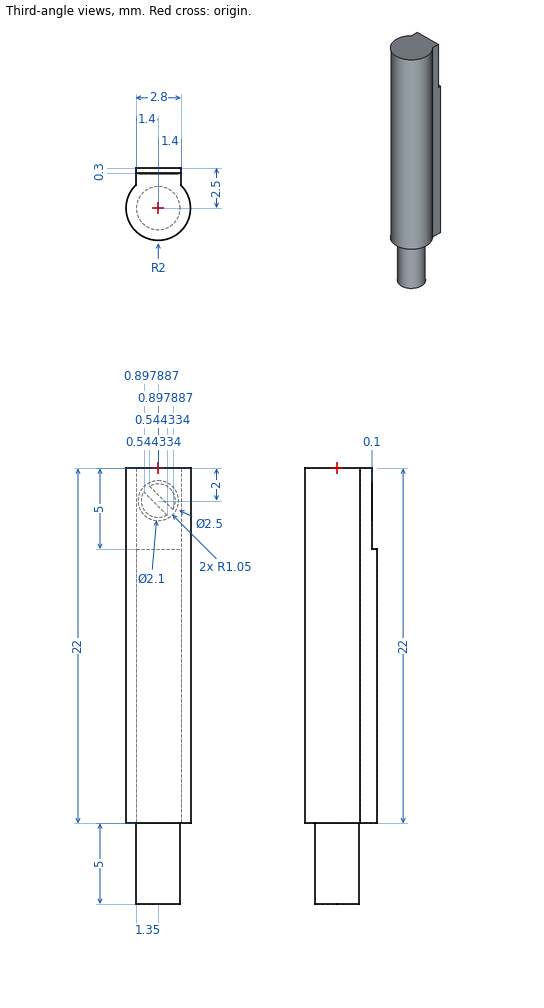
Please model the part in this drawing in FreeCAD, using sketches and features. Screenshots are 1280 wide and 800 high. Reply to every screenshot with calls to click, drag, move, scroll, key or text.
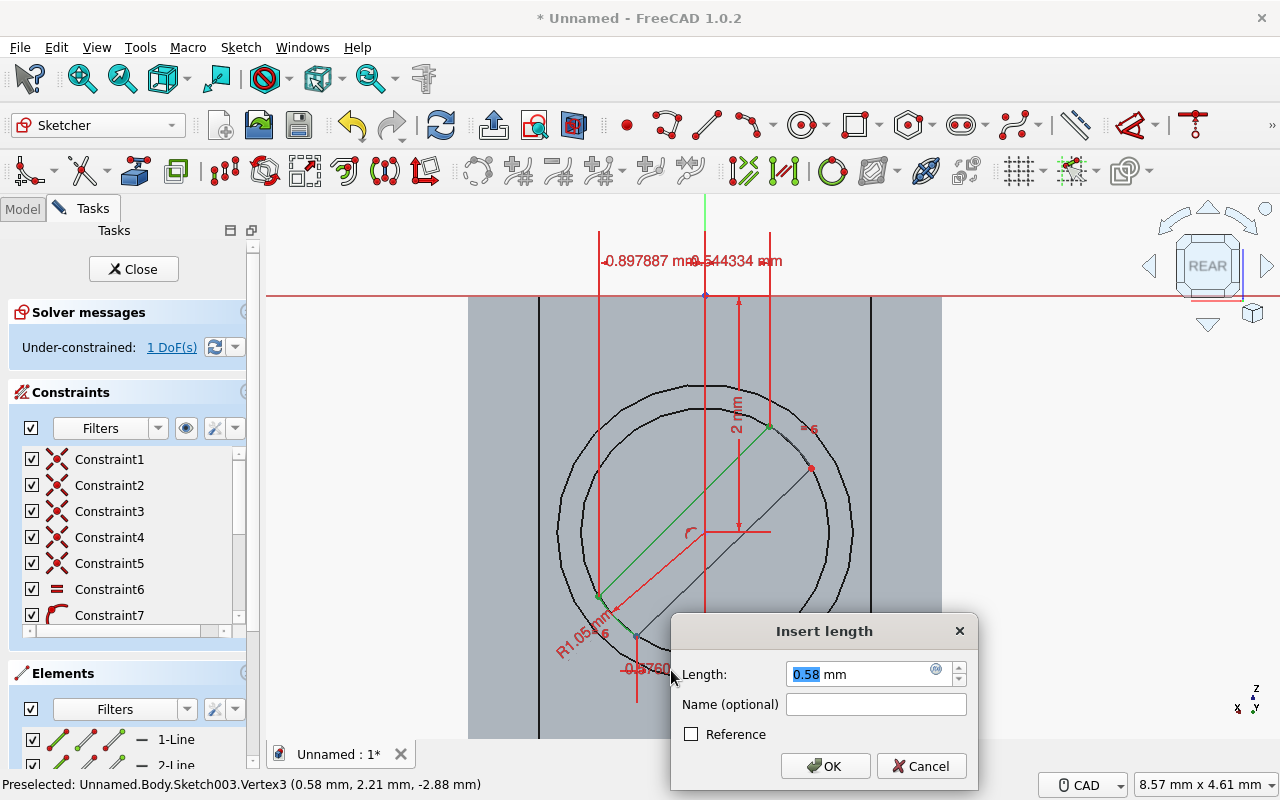
text(0.544334)
key(Return)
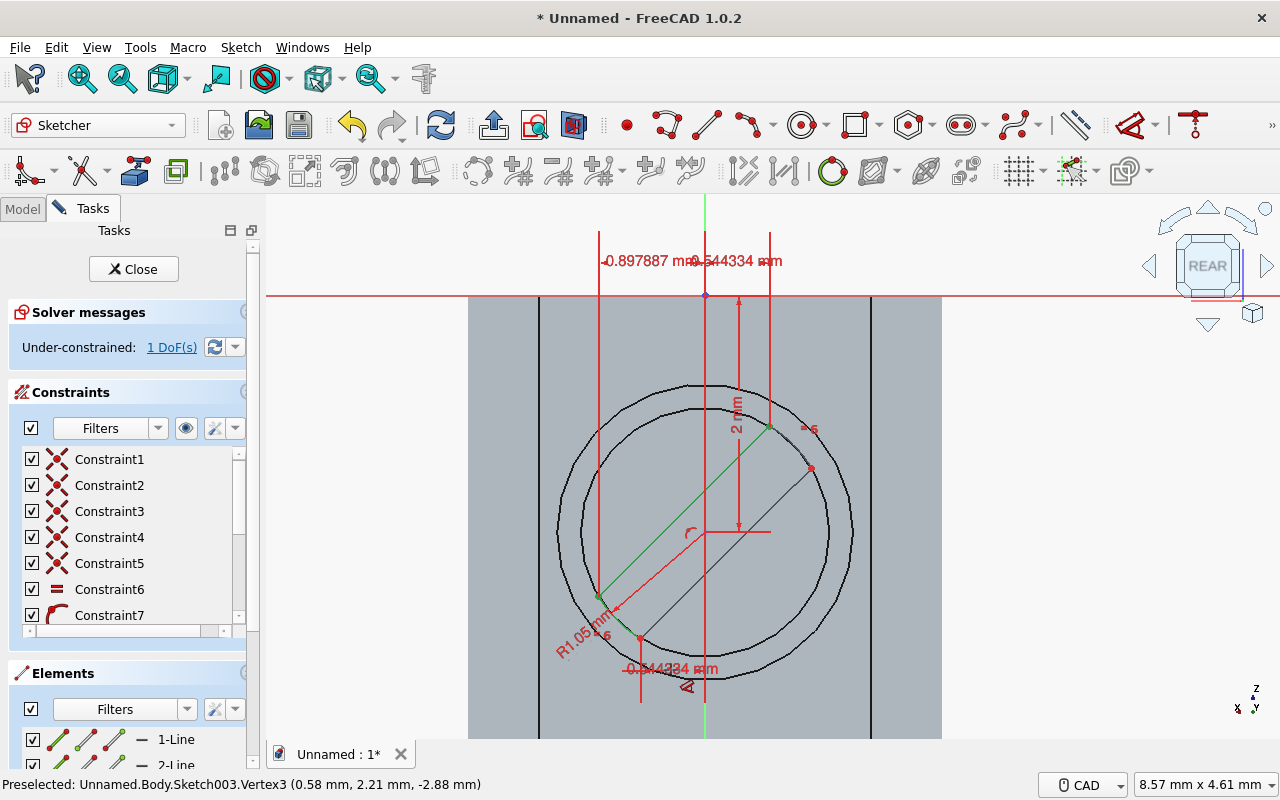
click(812, 468)
click(758, 502)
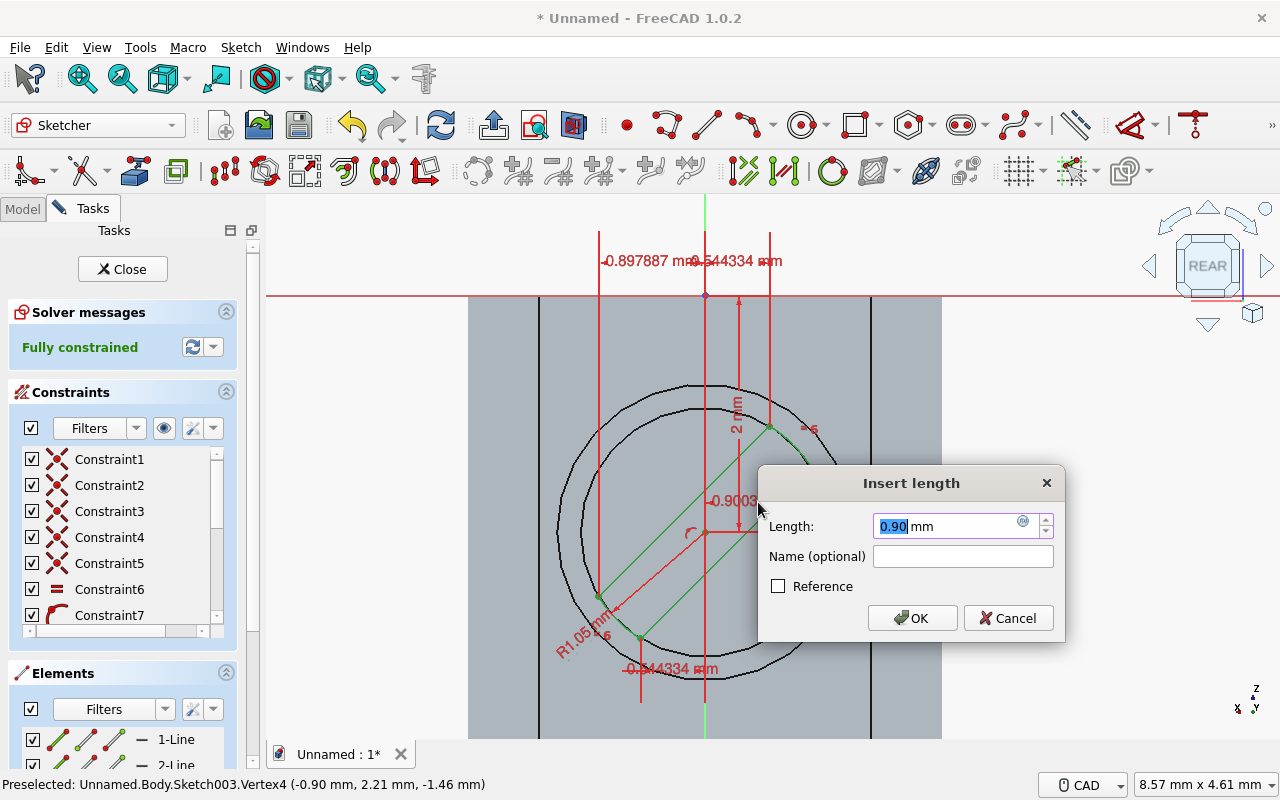
text(0.897887)
key(Return)
key(Escape)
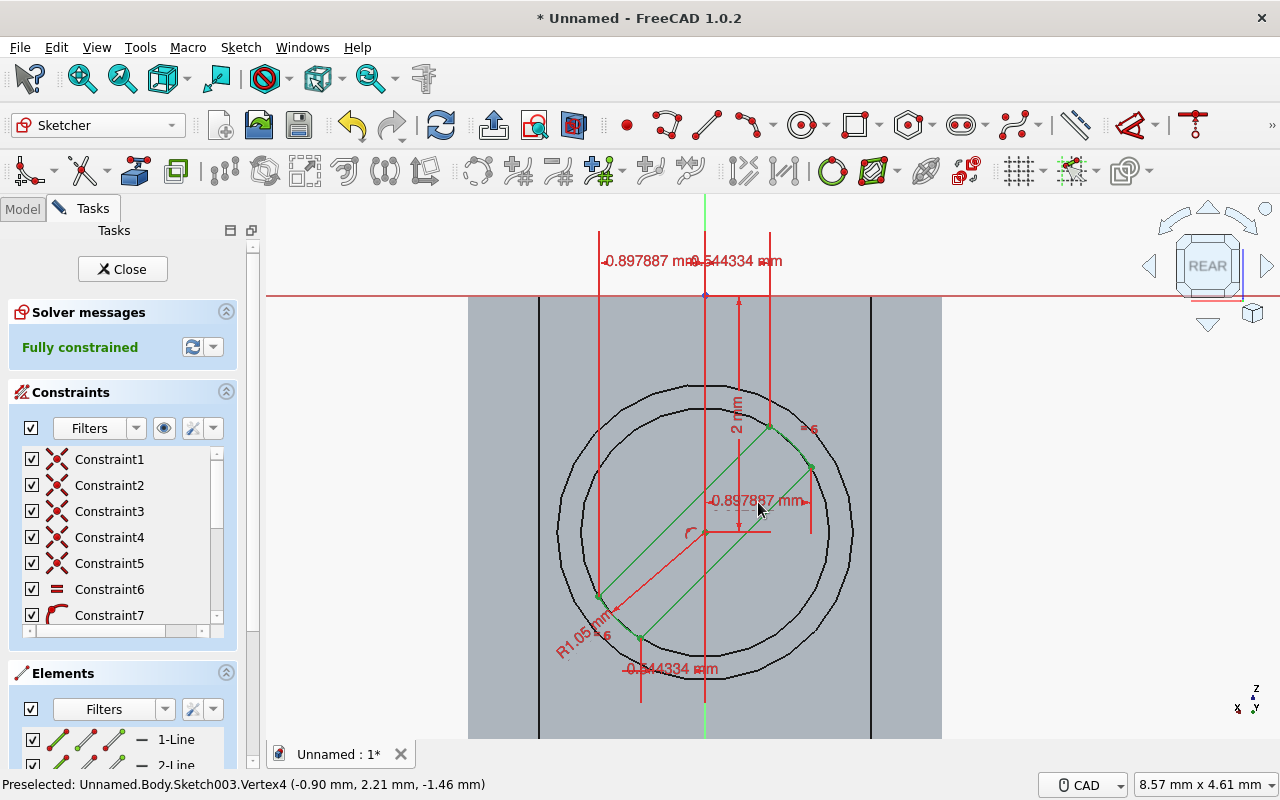
click(123, 269)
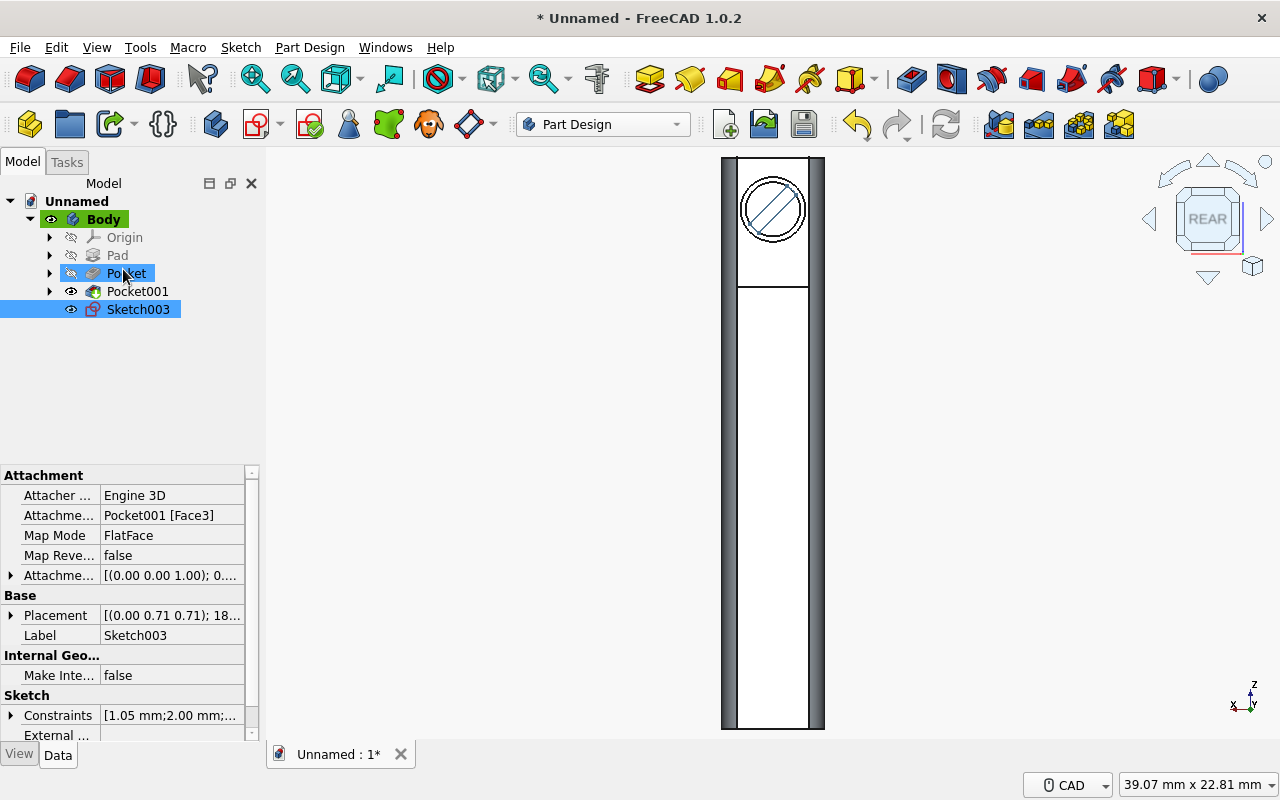
click(912, 80)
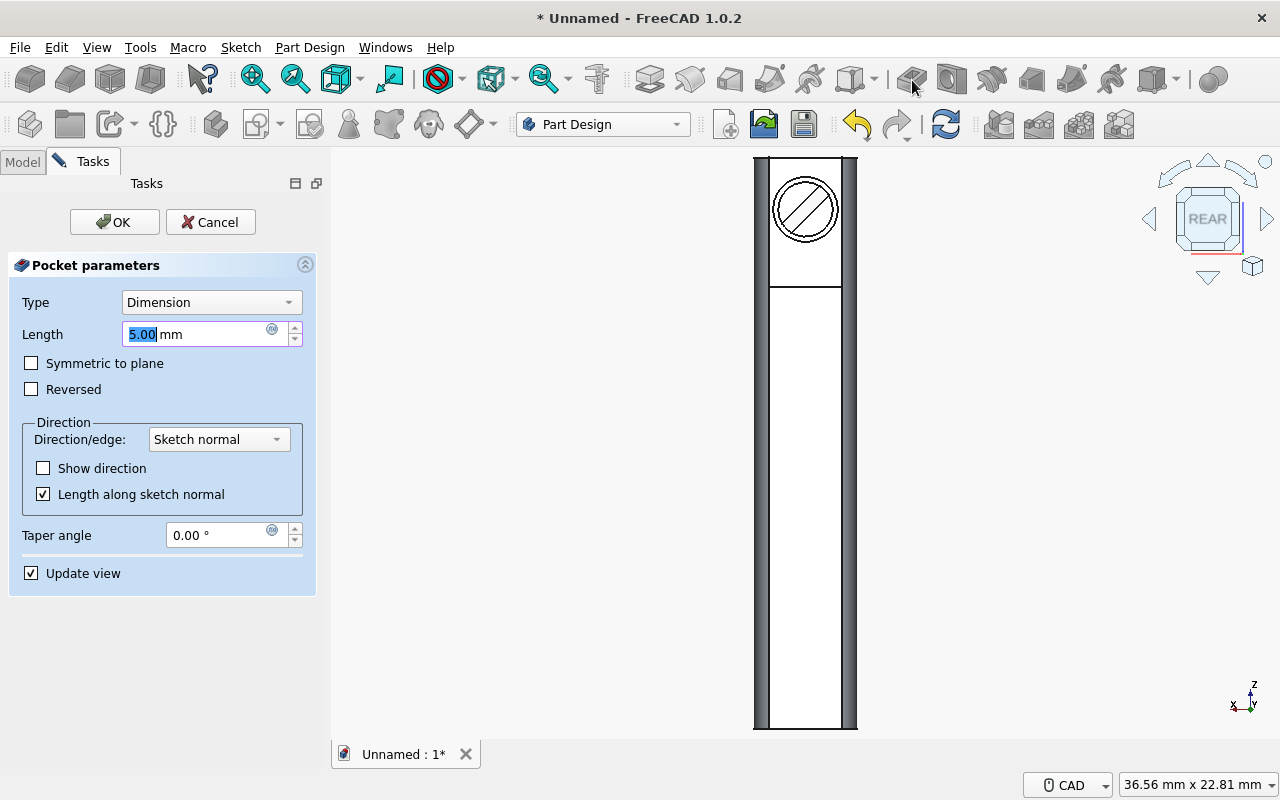
text(0.1)
key(Tab)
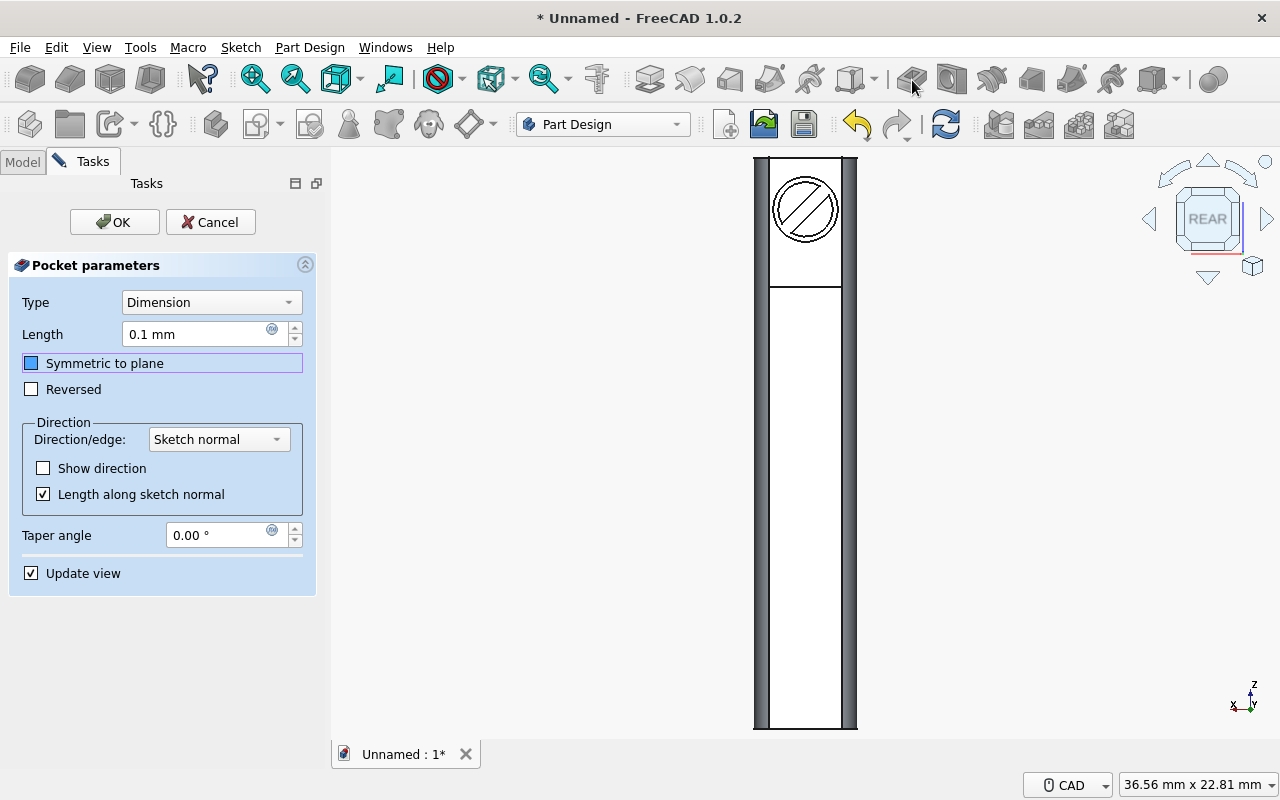
click(115, 222)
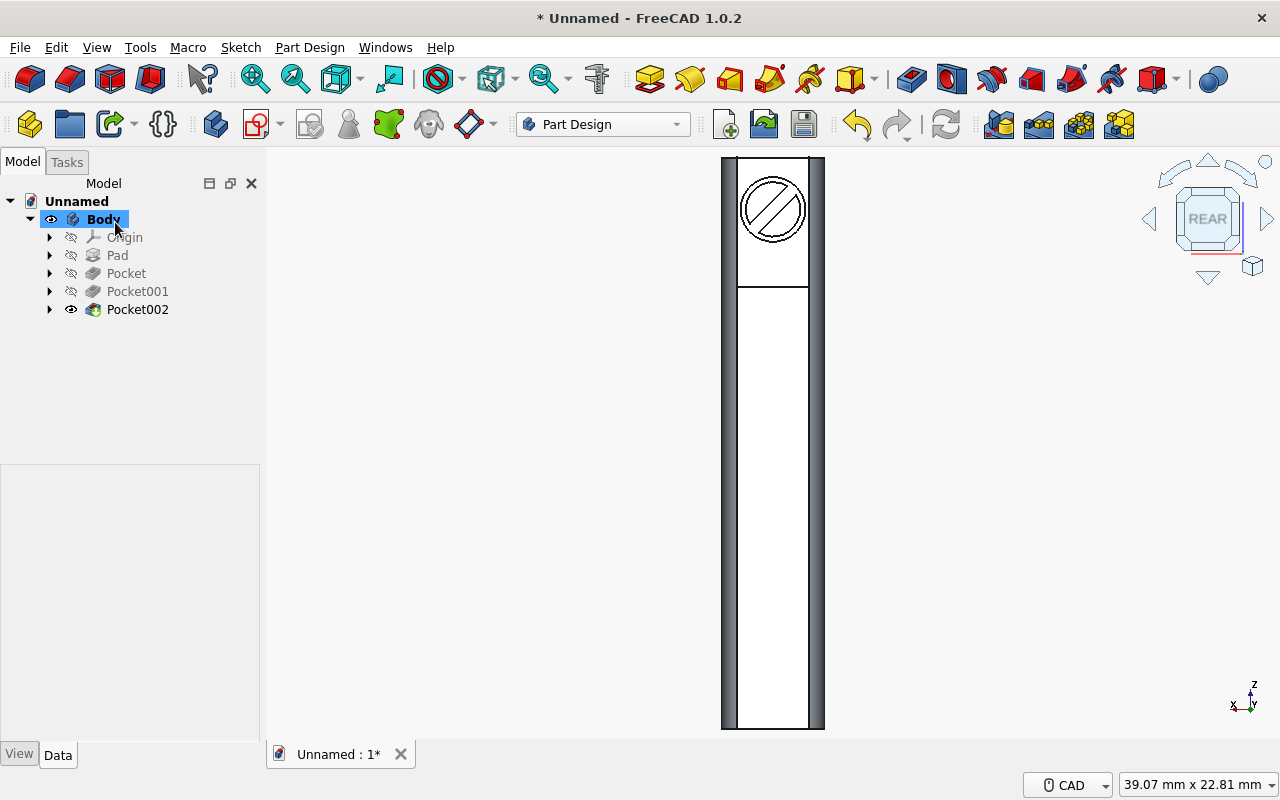
click(256, 124)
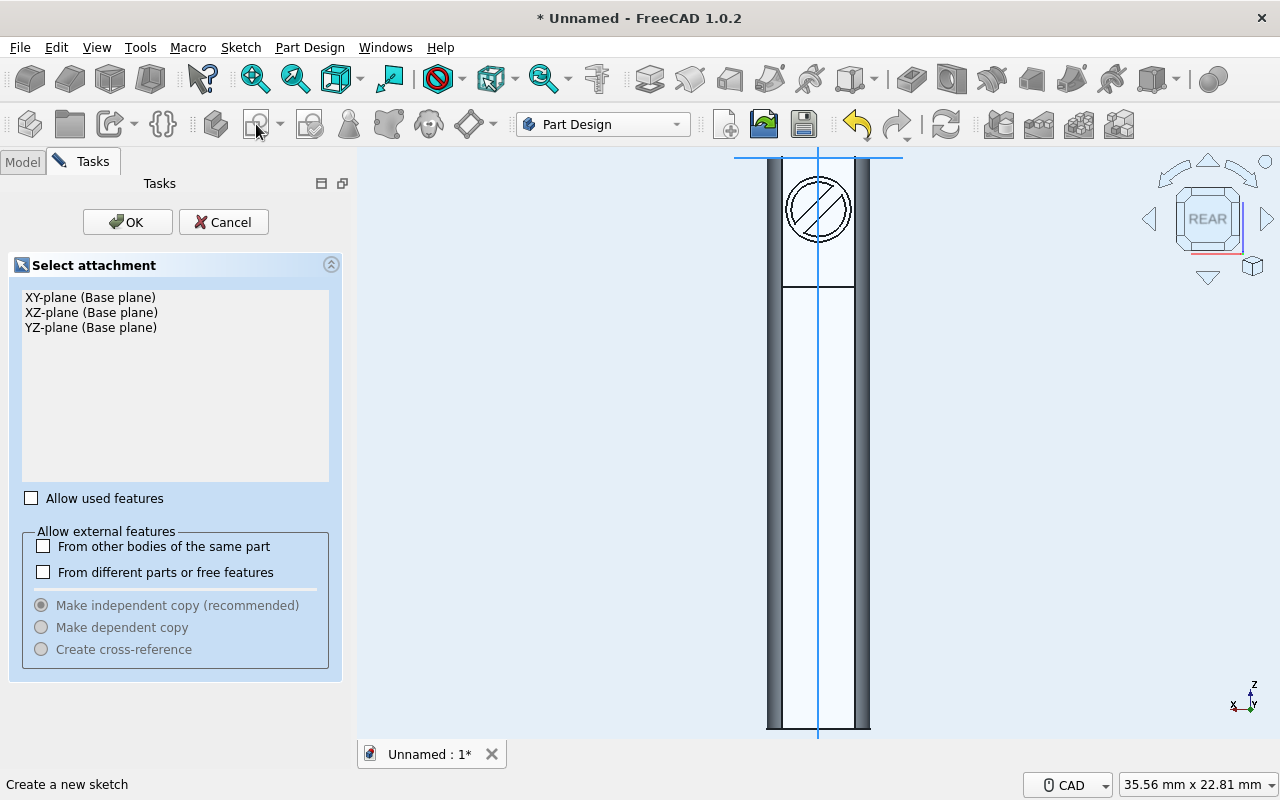
click(82, 312)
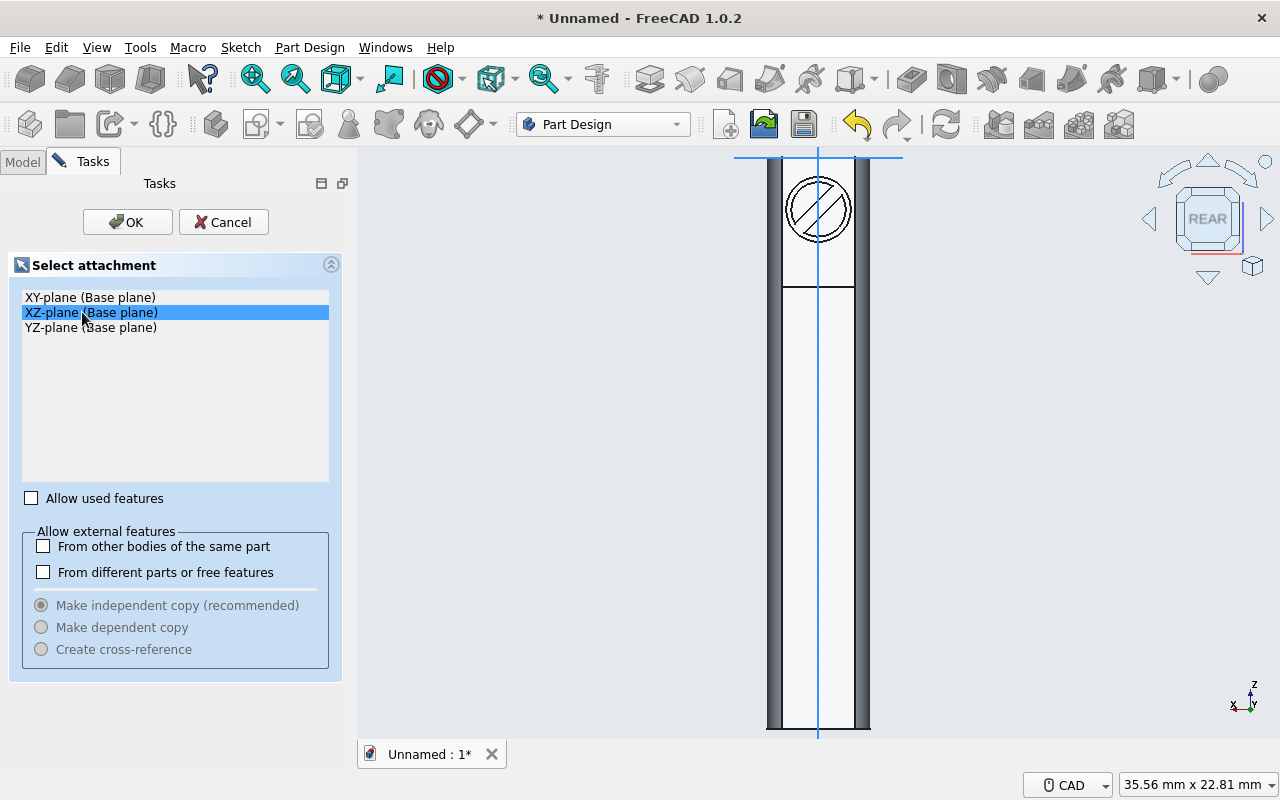
click(128, 222)